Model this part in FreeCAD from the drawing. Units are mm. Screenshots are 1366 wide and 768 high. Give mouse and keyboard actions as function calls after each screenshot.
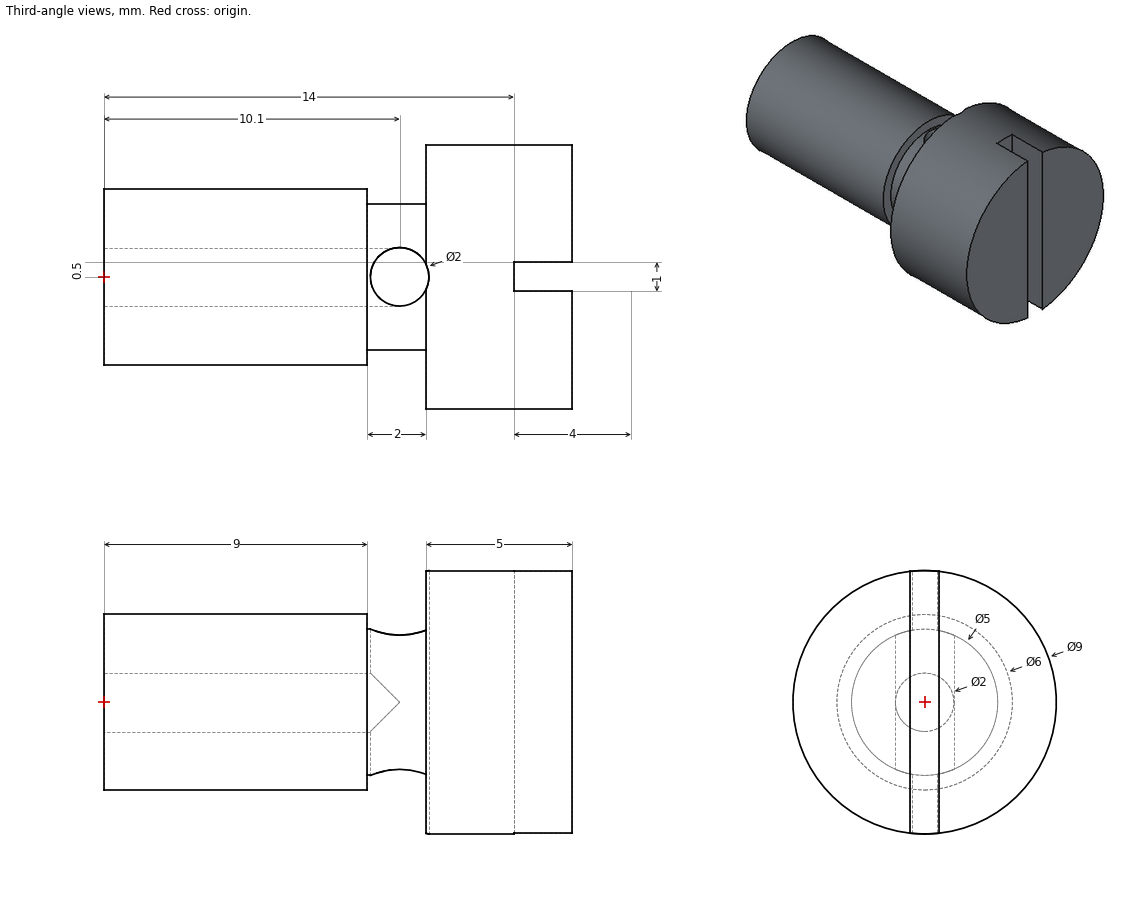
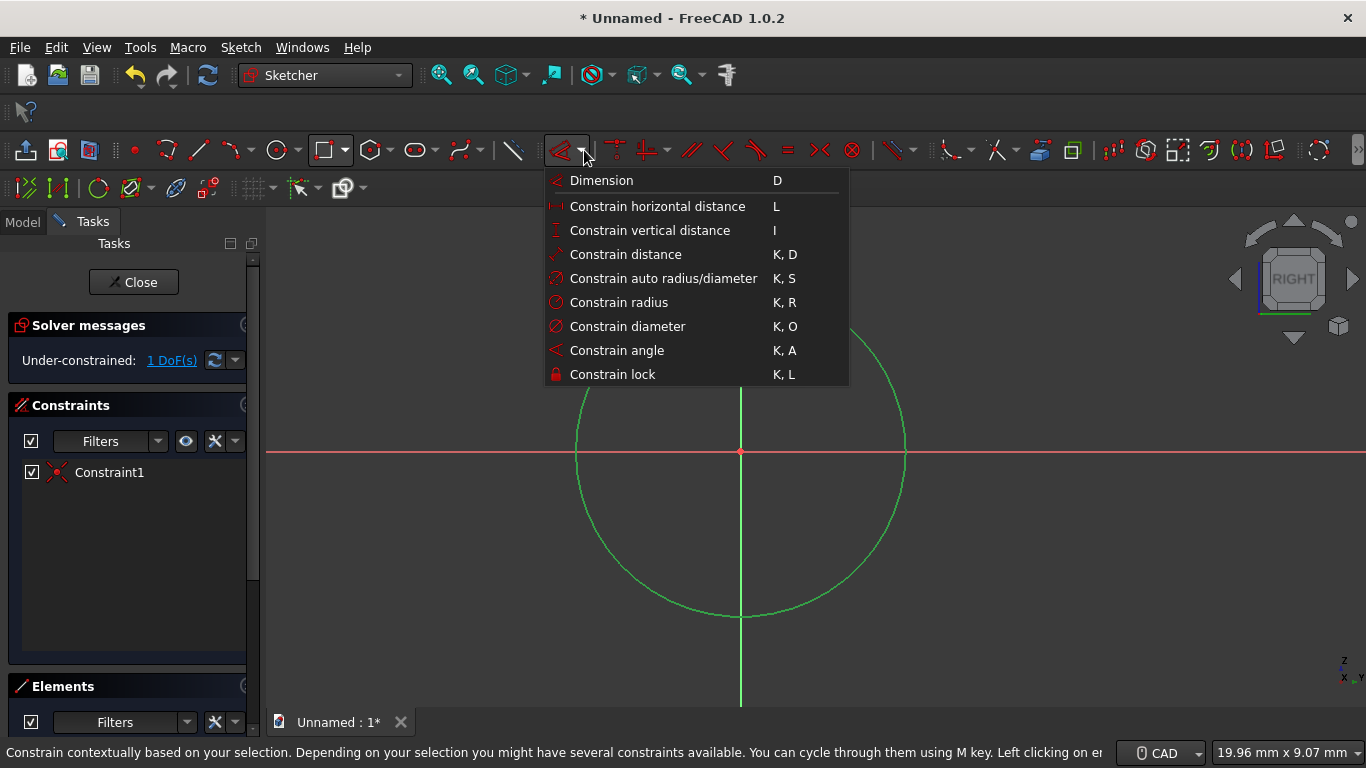
click(697, 326)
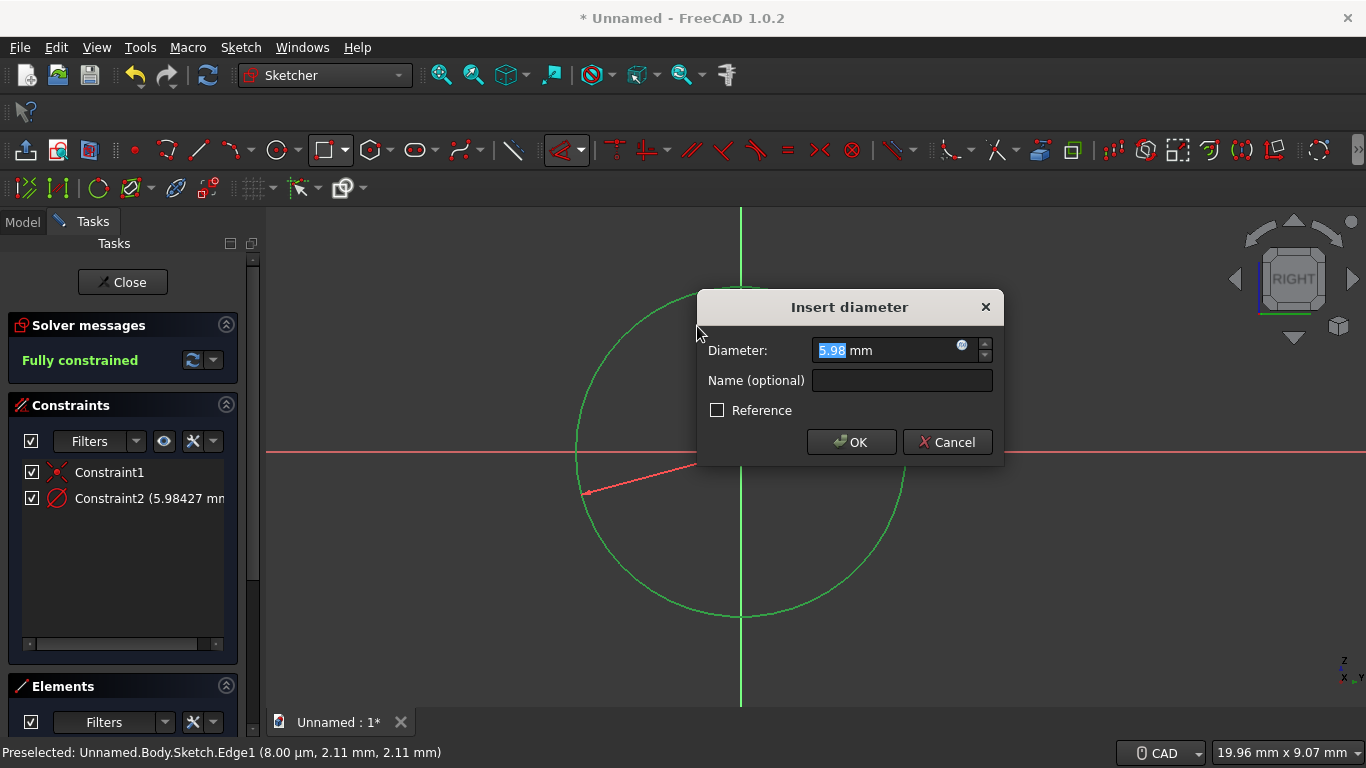
text(6)
key(Return)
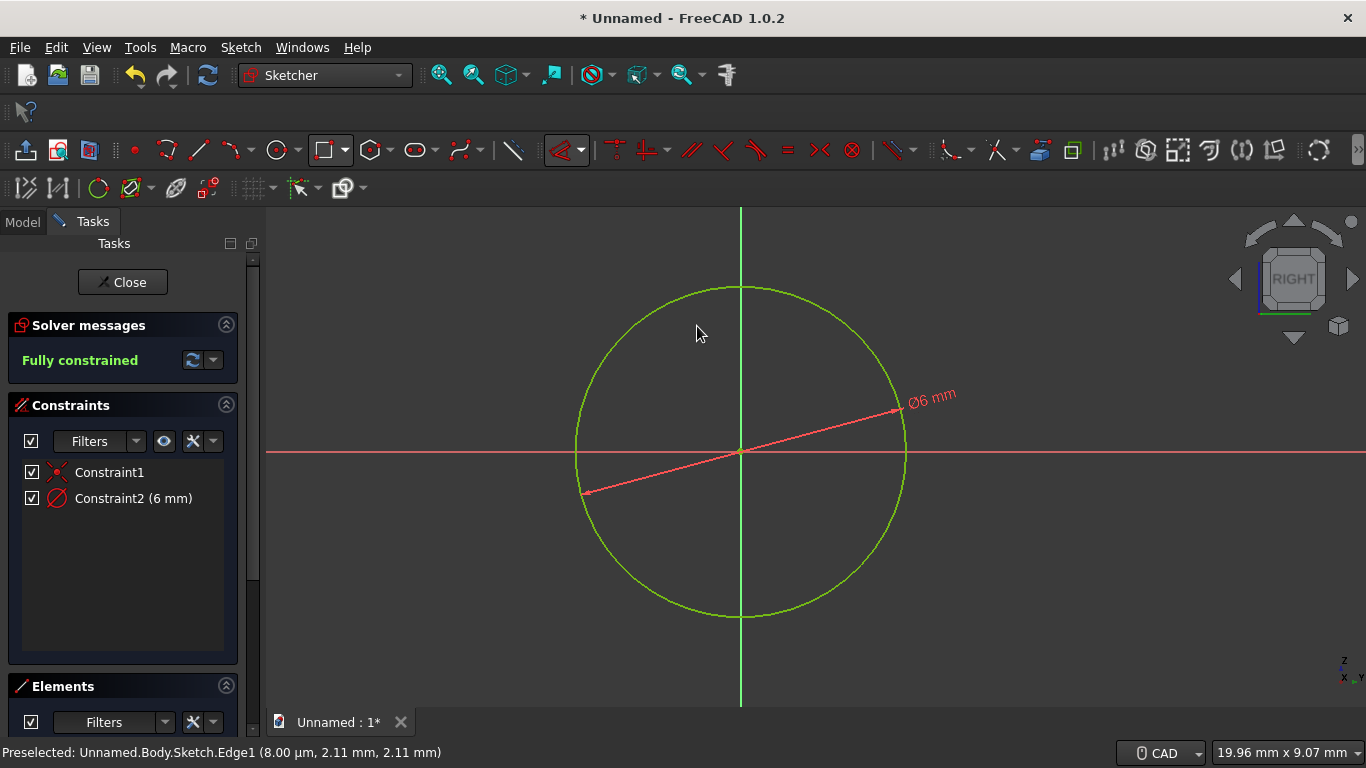
click(123, 282)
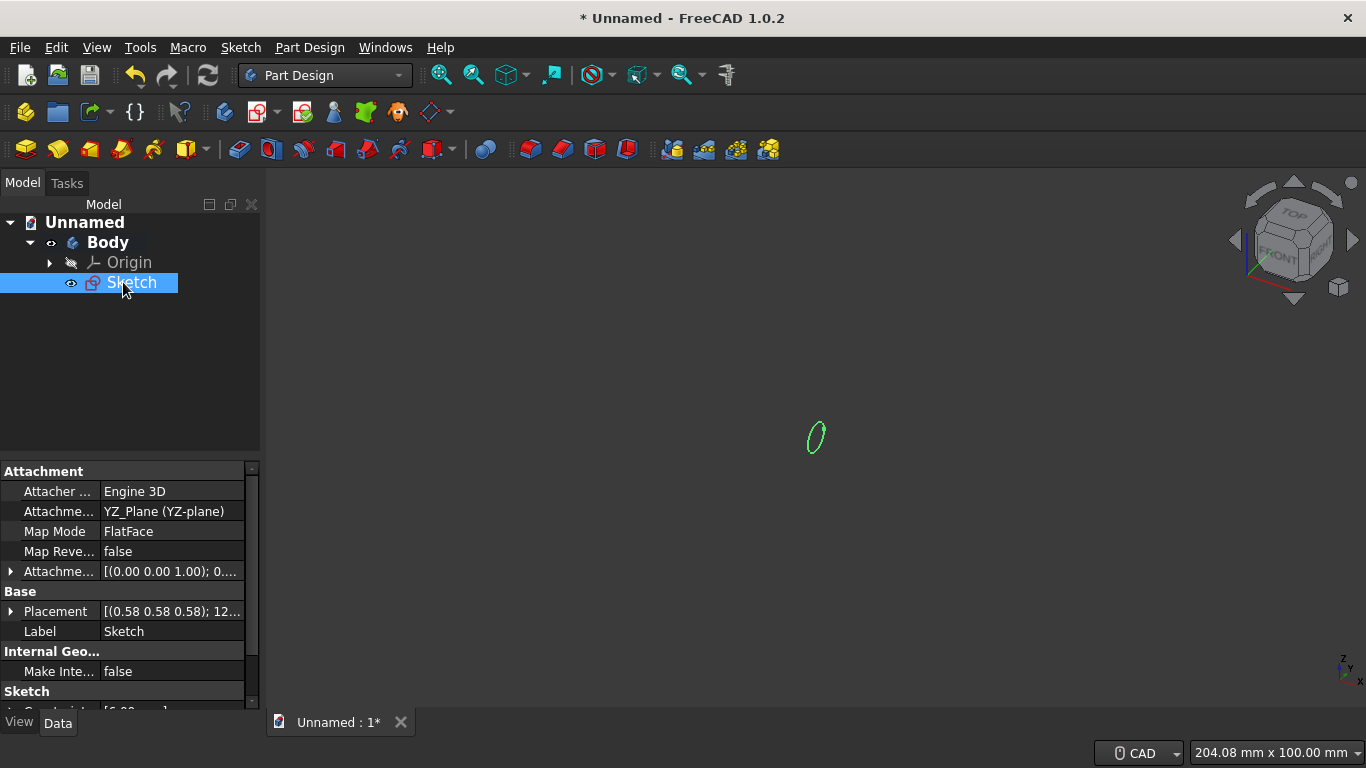
click(26, 150)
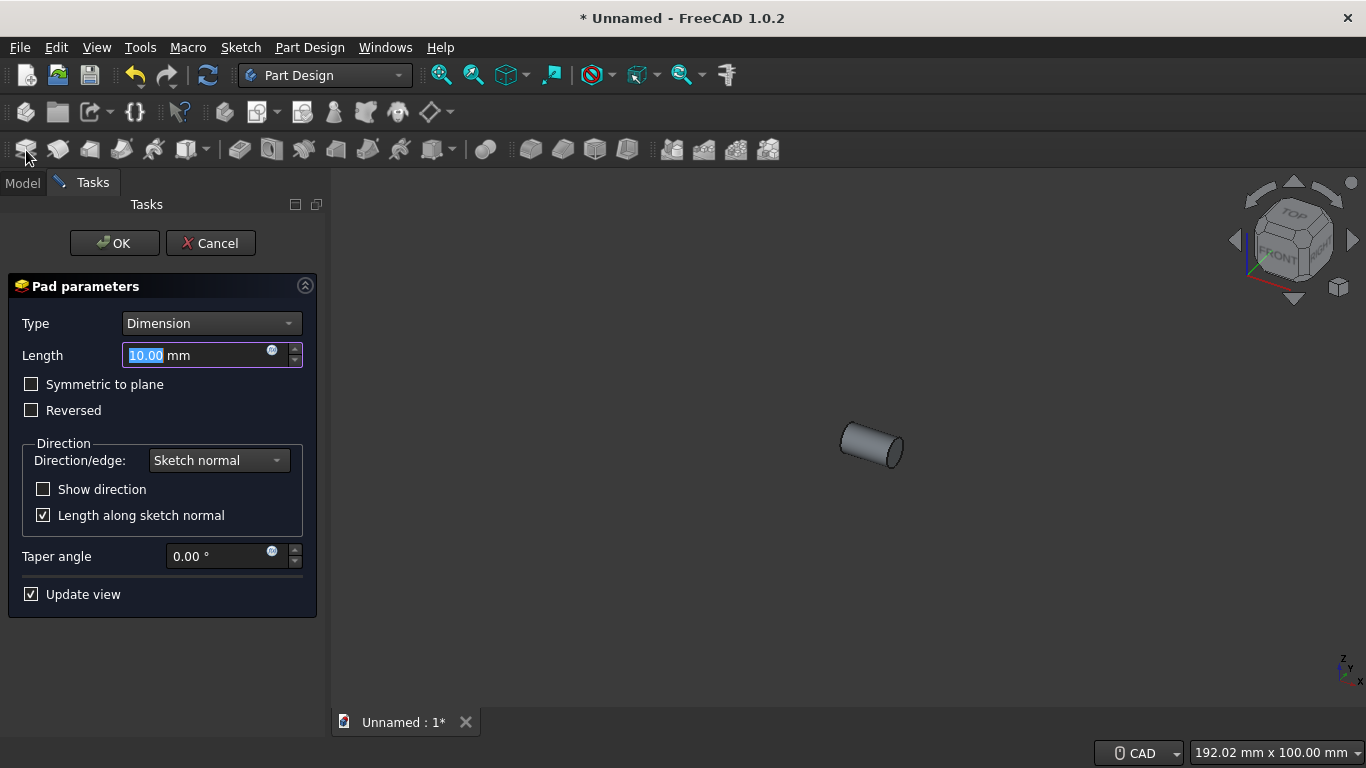
text(9)
key(Tab)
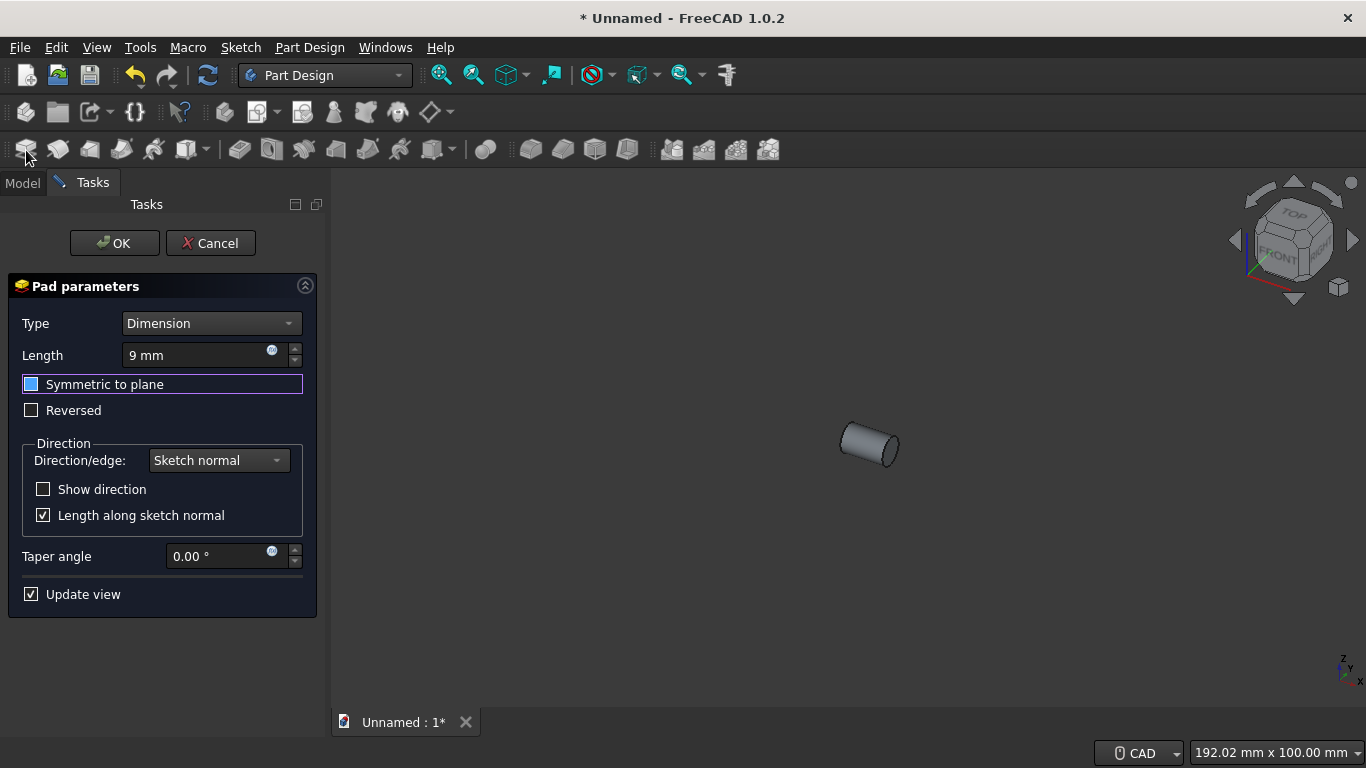
click(115, 243)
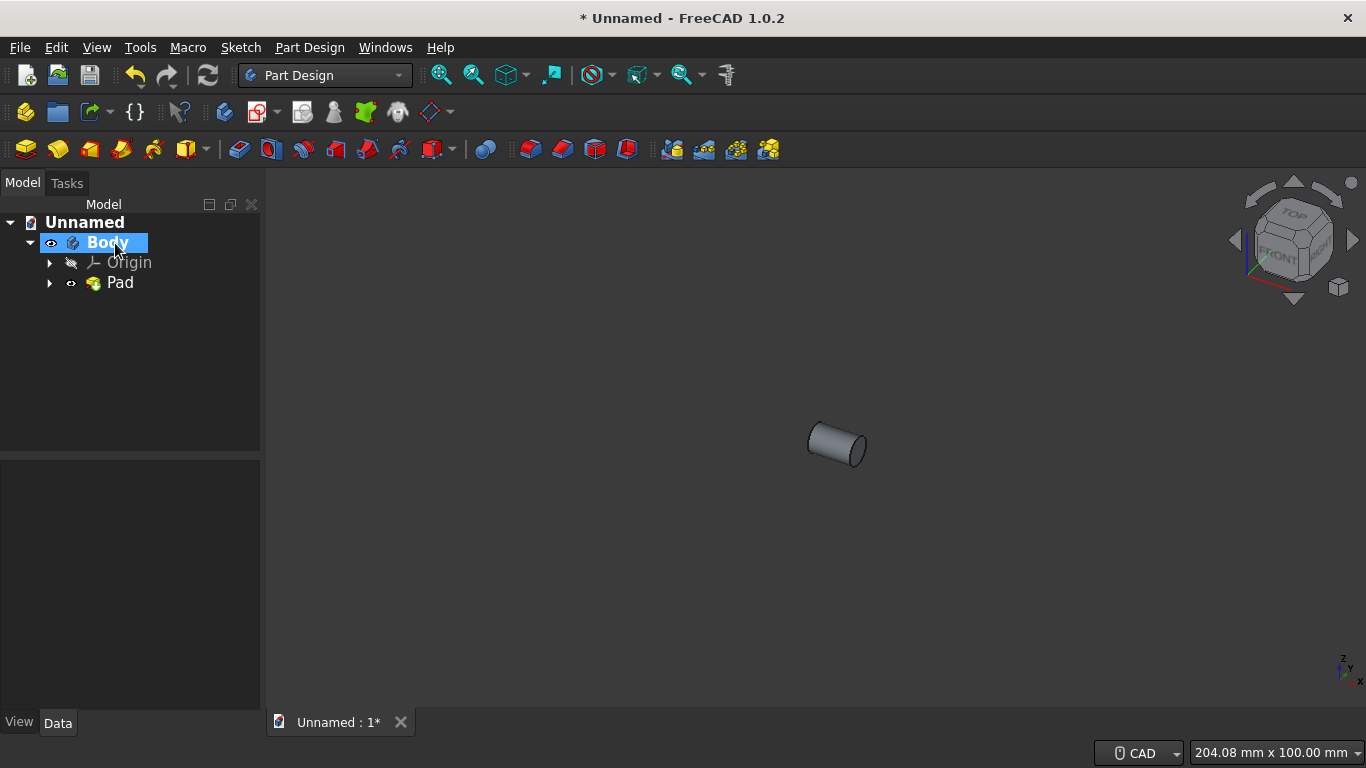
click(442, 76)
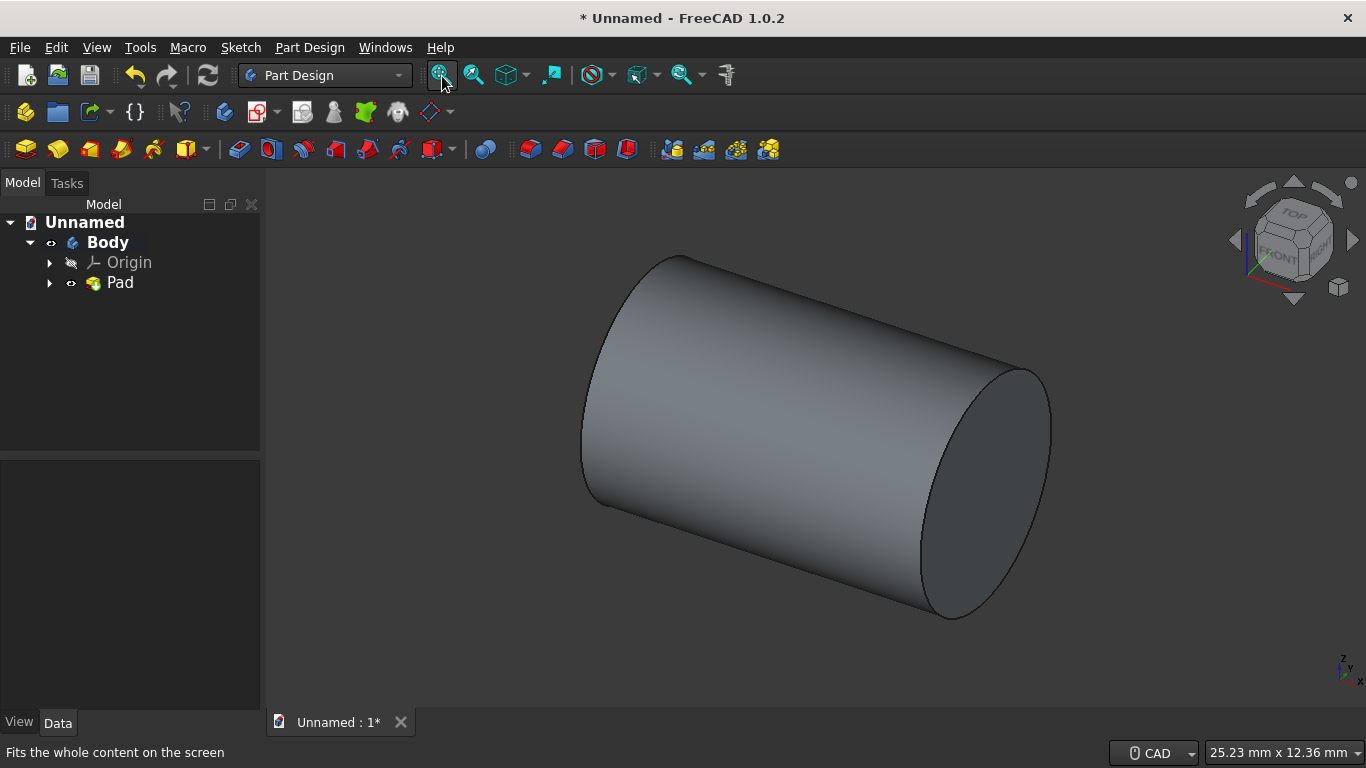
click(986, 493)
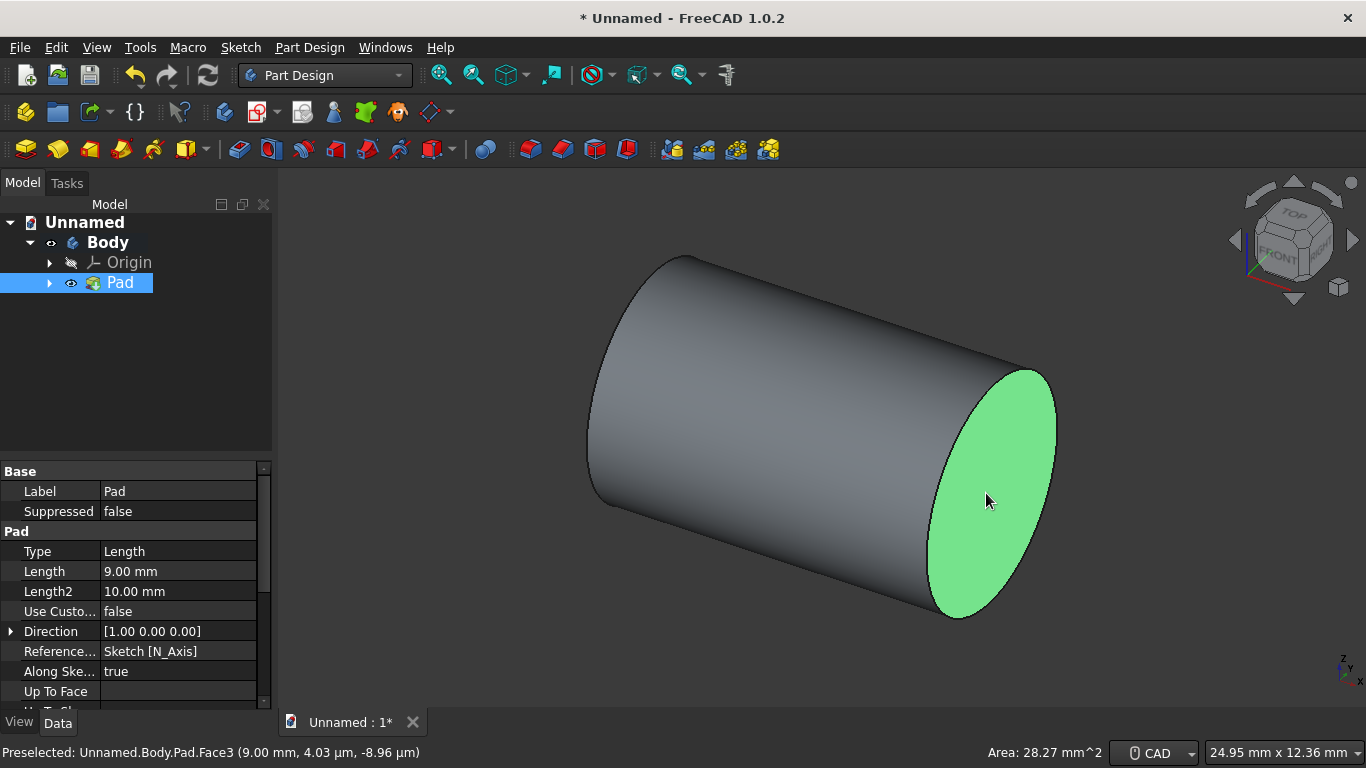
click(258, 112)